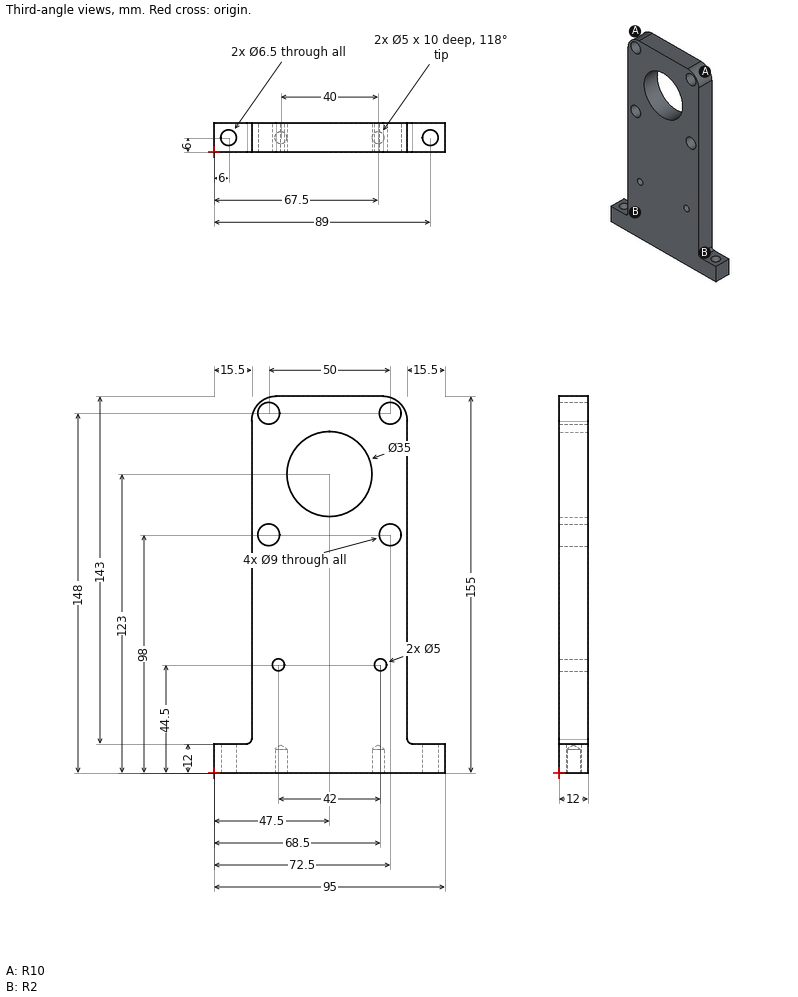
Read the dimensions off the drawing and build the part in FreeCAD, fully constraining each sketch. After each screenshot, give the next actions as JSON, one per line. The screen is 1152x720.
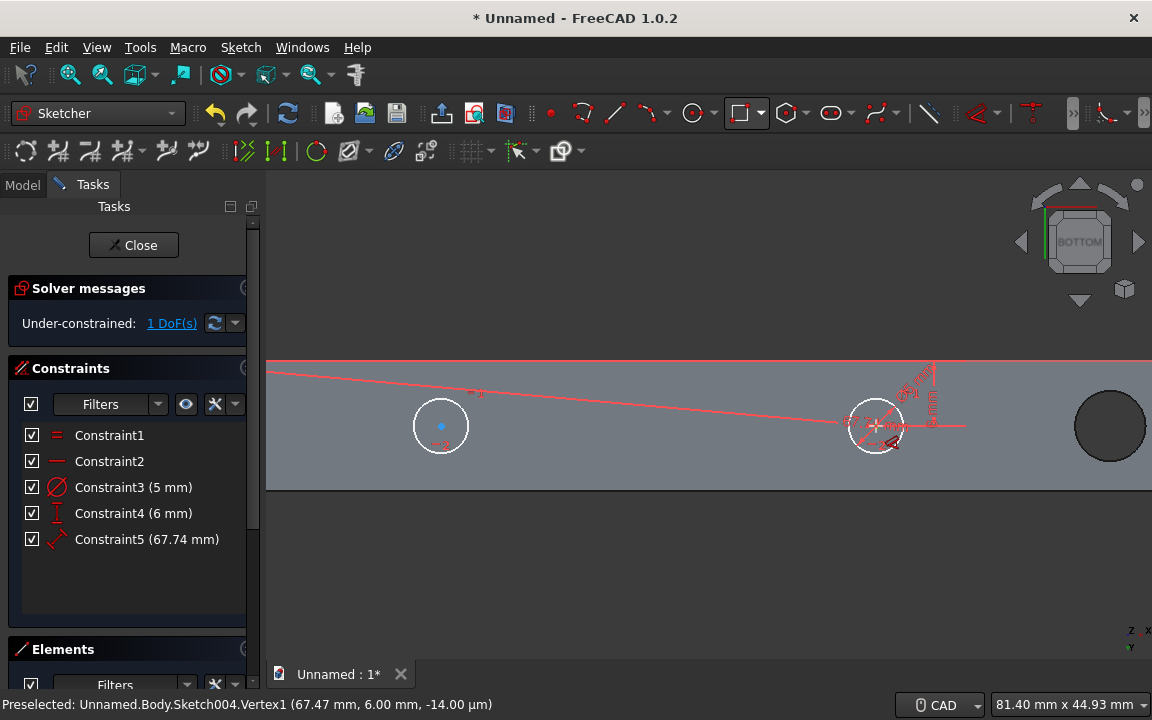
{"action": "left_click", "coordinate": [441, 426]}
{"action": "left_click", "coordinate": [659, 460]}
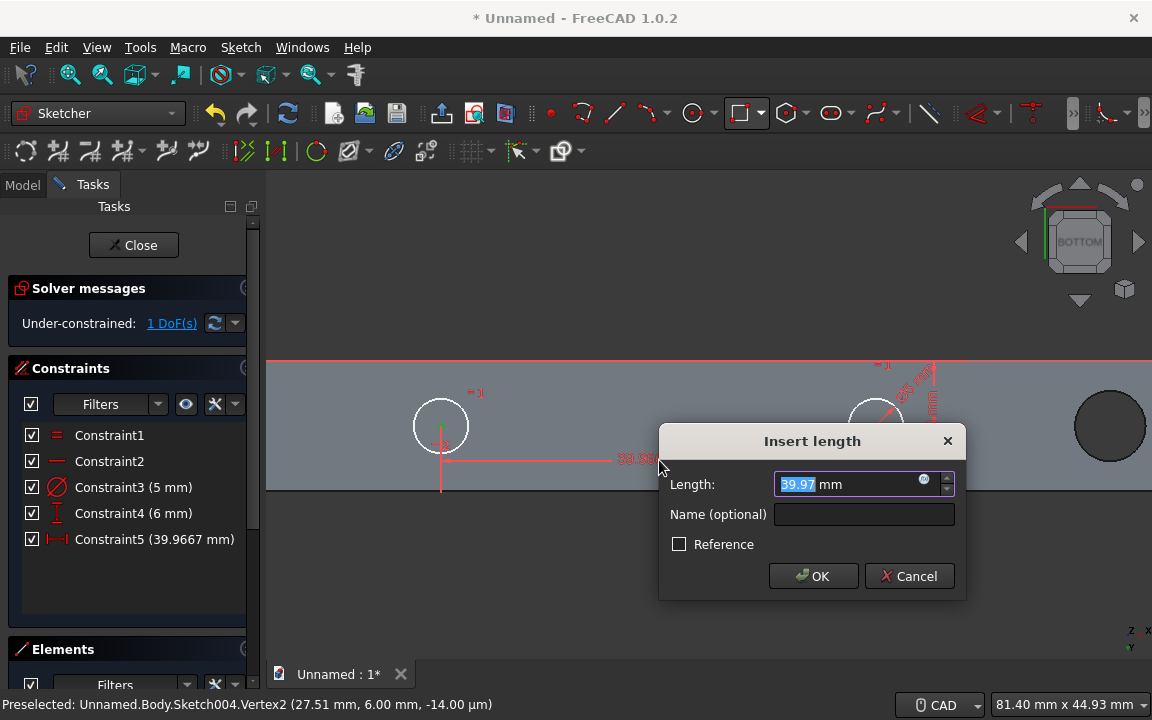
{"action": "type", "text": "40"}
{"action": "key", "text": "Return"}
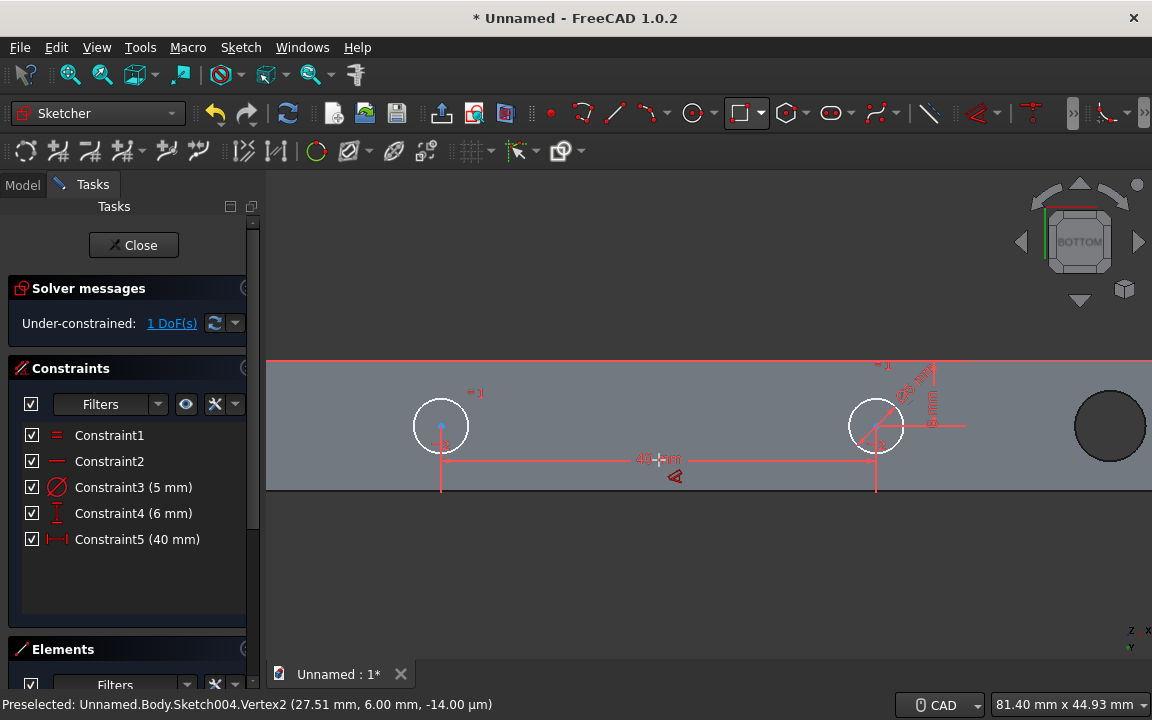
{"action": "left_click", "coordinate": [876, 426]}
{"action": "left_click", "coordinate": [585, 327]}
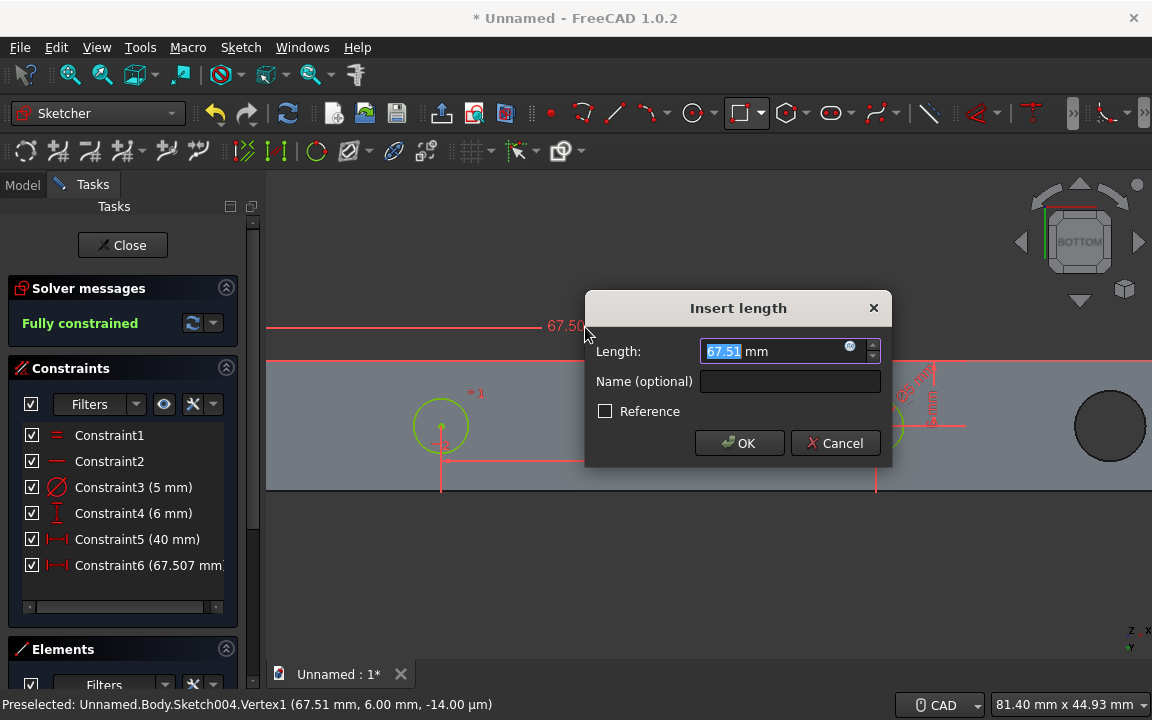
{"action": "type", "text": "67.5"}
{"action": "key", "text": "Return"}
{"action": "key", "text": "Escape"}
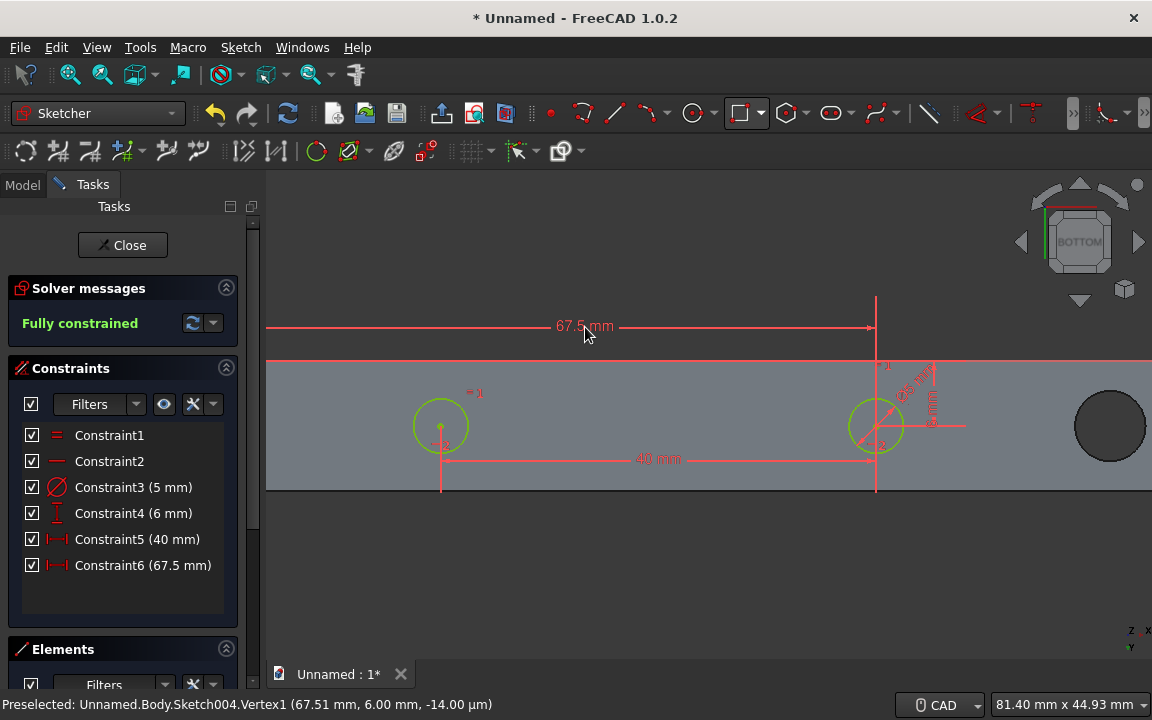
{"action": "left_click", "coordinate": [123, 245]}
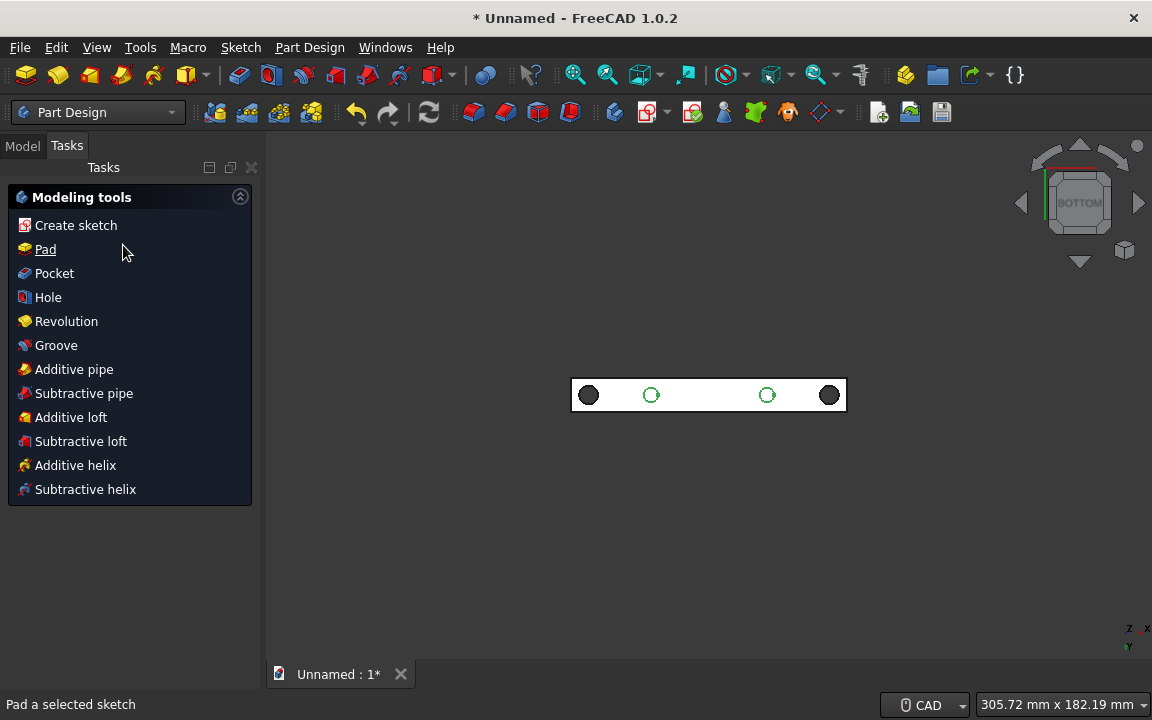
{"action": "left_click", "coordinate": [272, 76]}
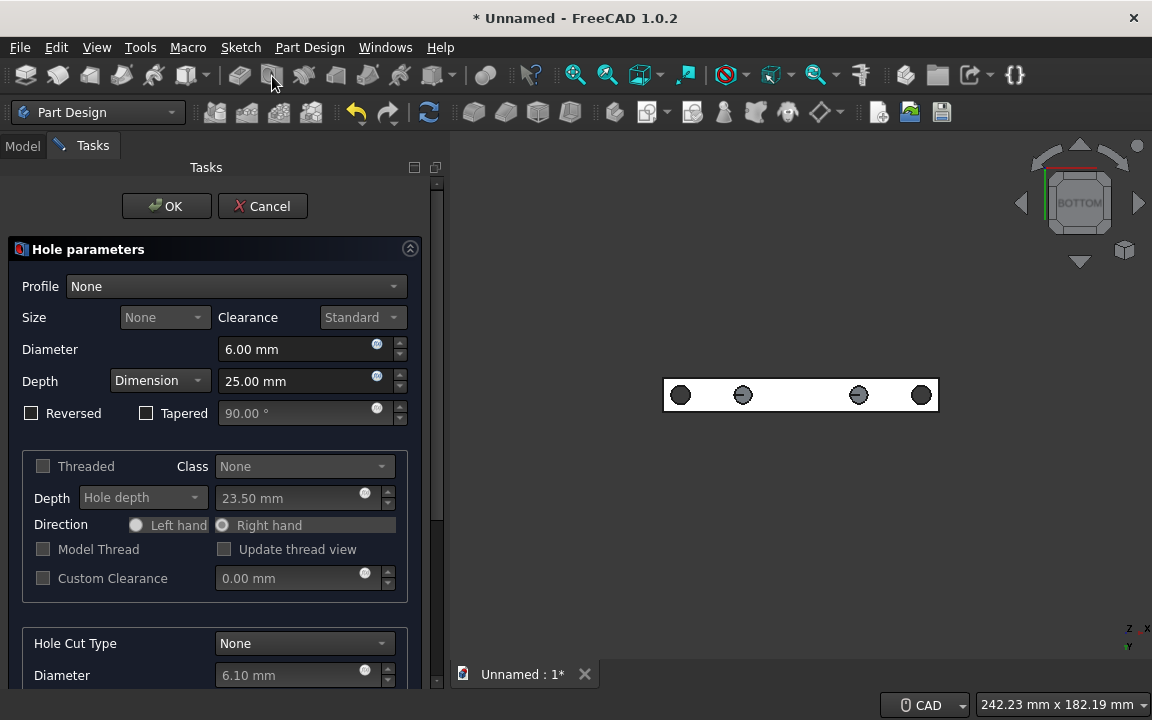
{"action": "triple_click", "coordinate": [305, 349]}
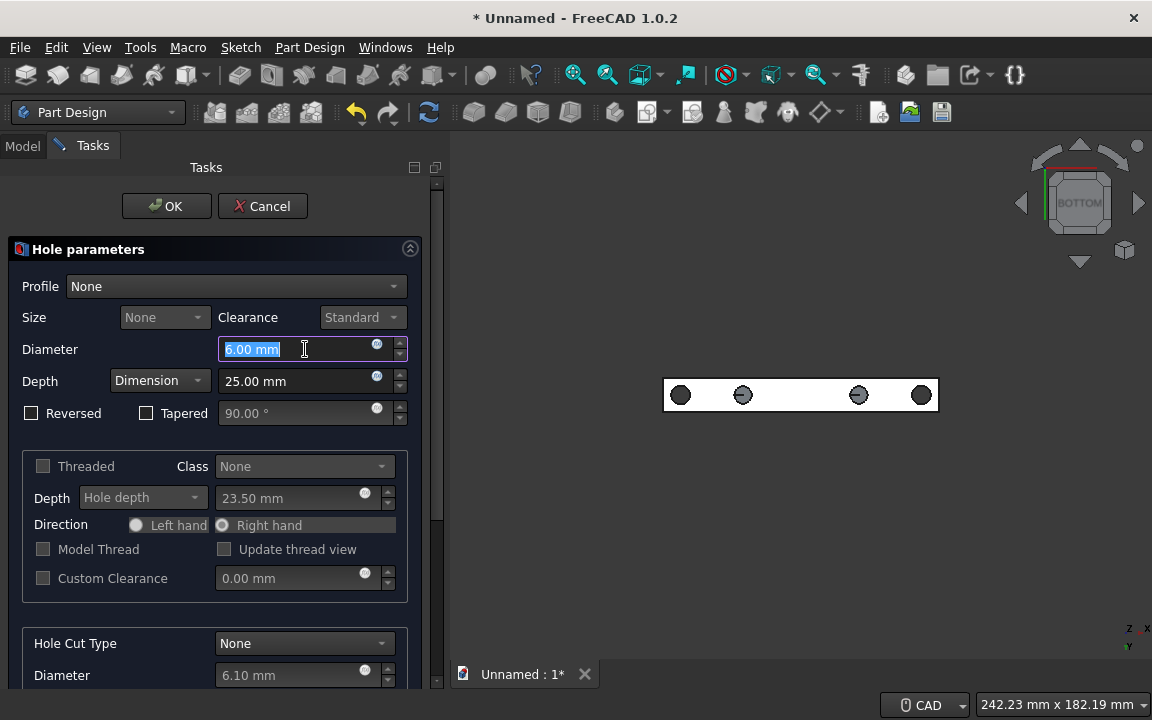
{"action": "type", "text": "5"}
{"action": "key", "text": "Tab"}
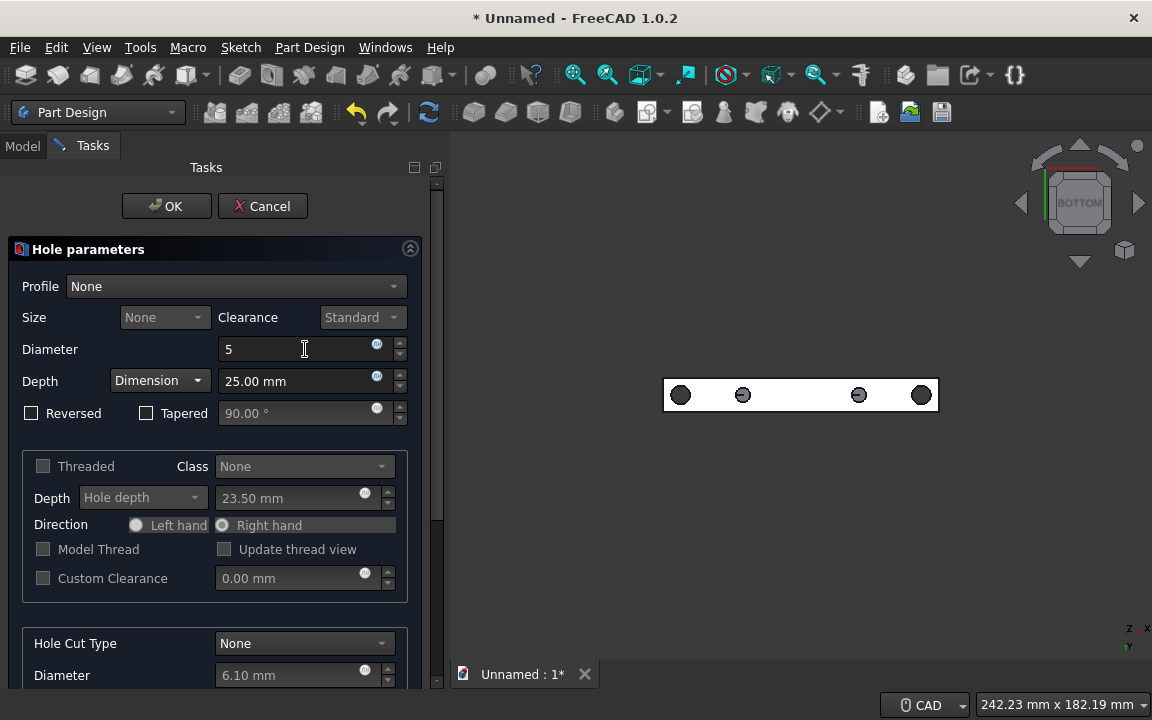
{"action": "triple_click", "coordinate": [305, 381]}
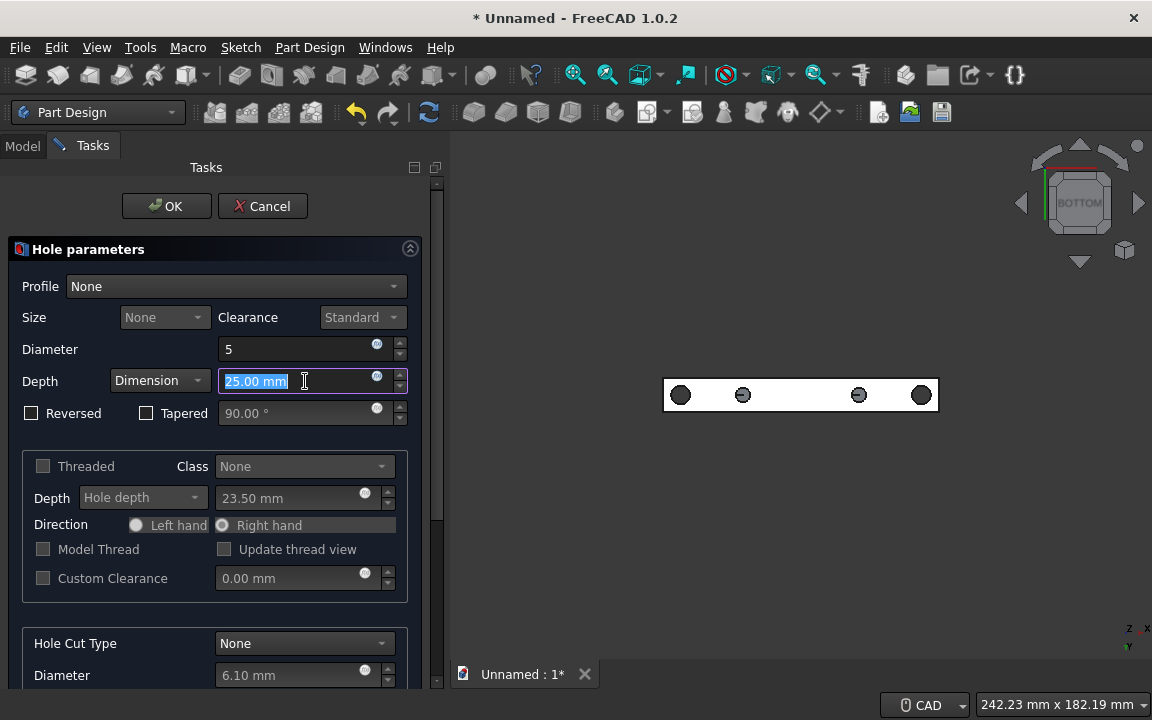
{"action": "type", "text": "10"}
{"action": "key", "text": "Tab"}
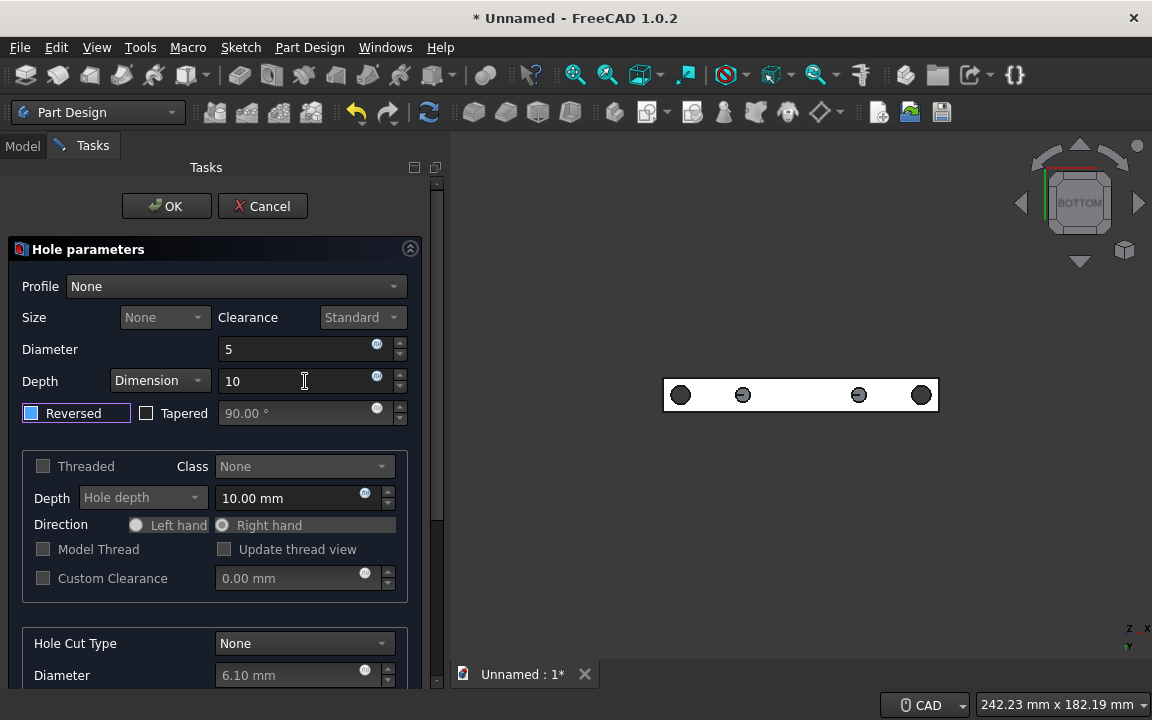
{"action": "left_click", "coordinate": [167, 206]}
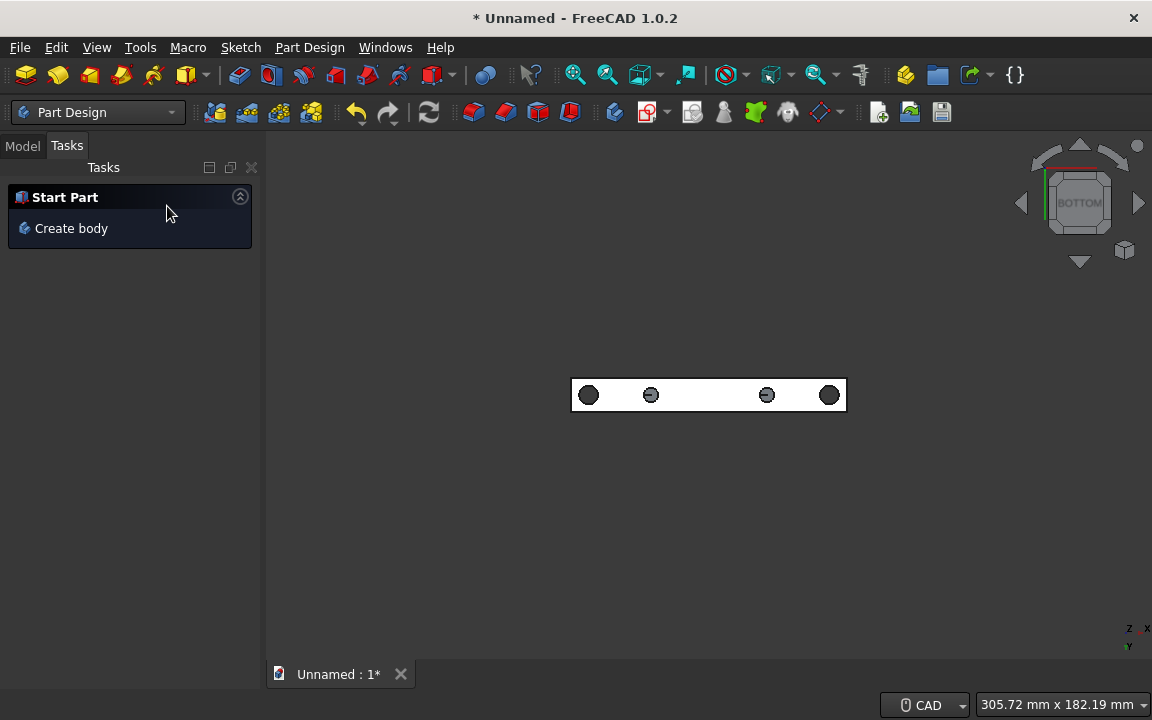
{"action": "key", "text": "v f"}